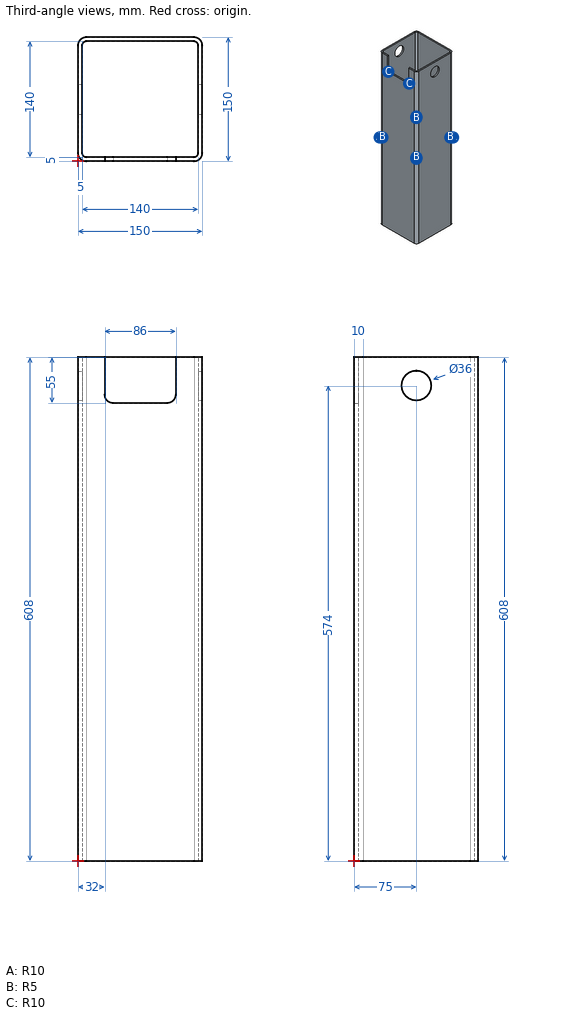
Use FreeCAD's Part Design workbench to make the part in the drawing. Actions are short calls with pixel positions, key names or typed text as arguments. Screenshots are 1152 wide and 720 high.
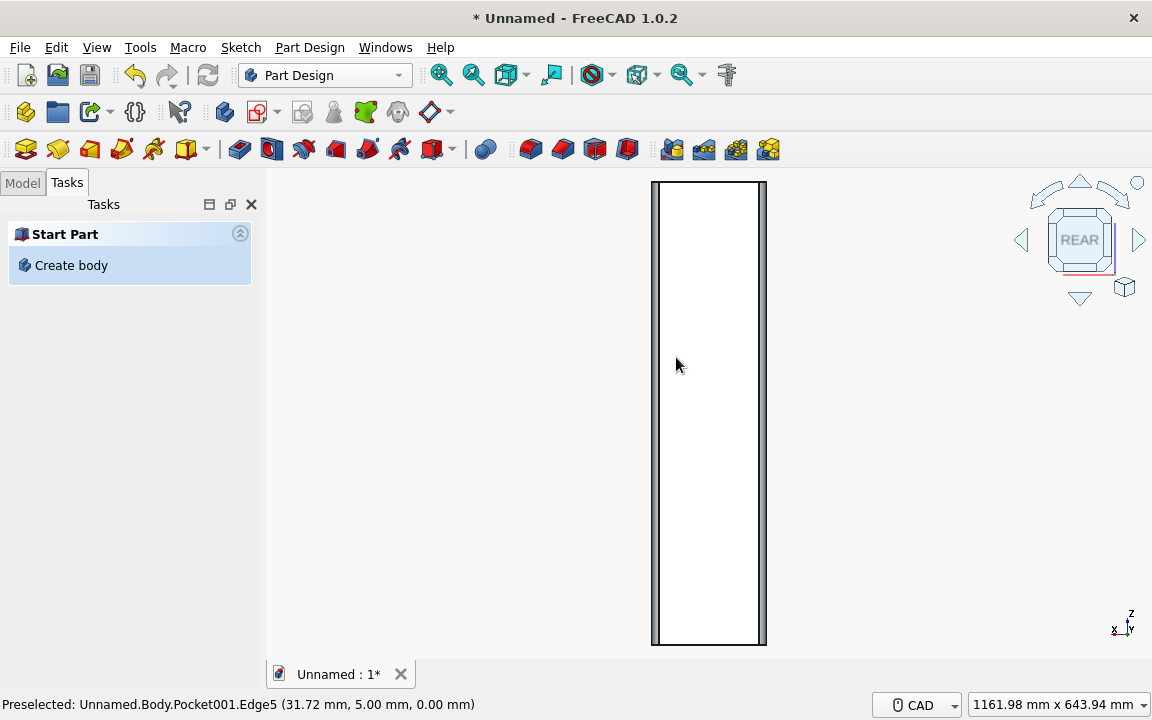
scroll(742, 223, up, 12)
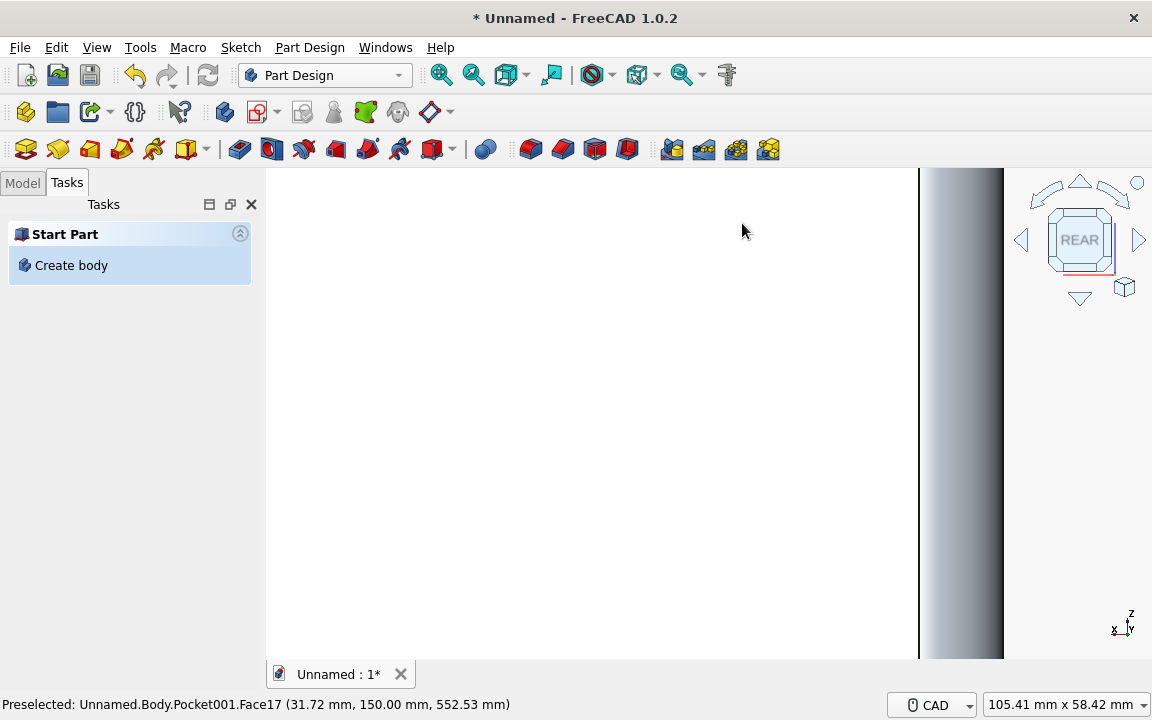
key(v)
key(f)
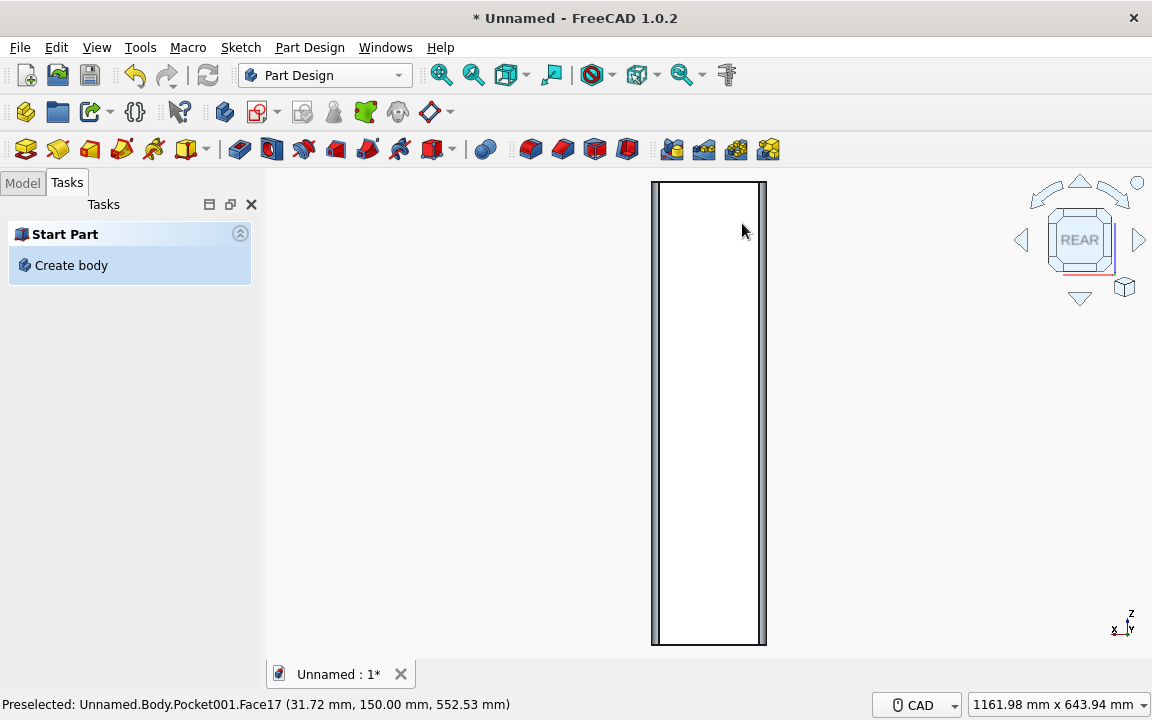
key(6)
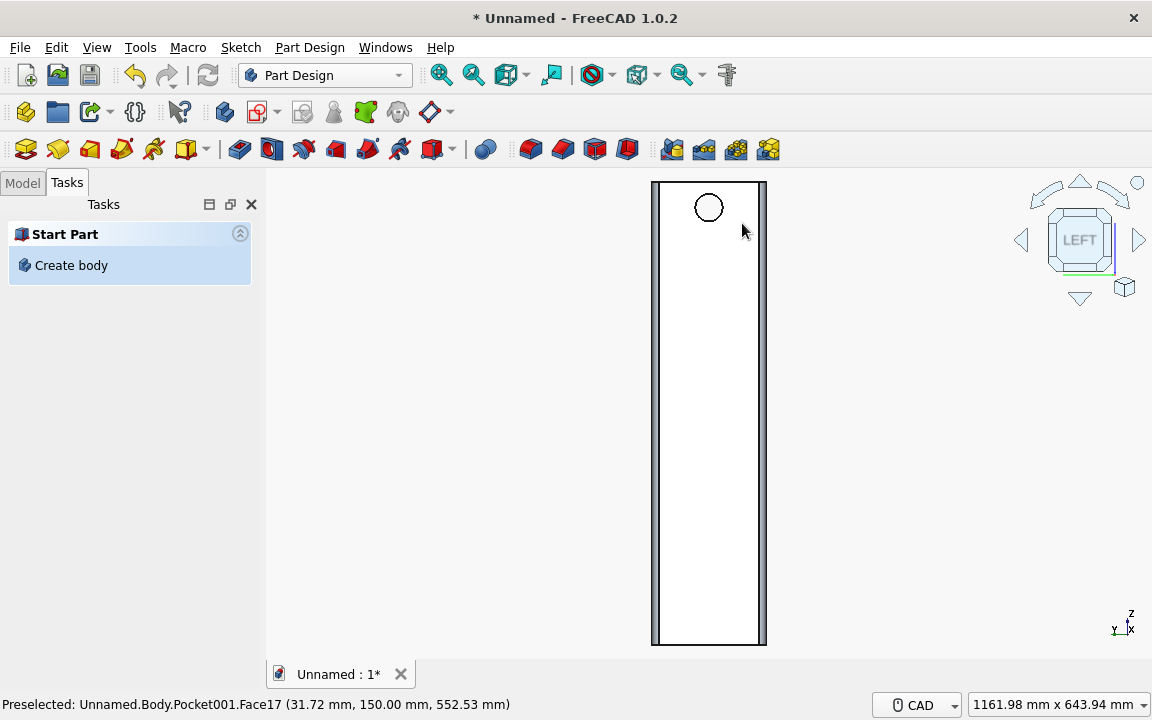
scroll(764, 223, up, 12)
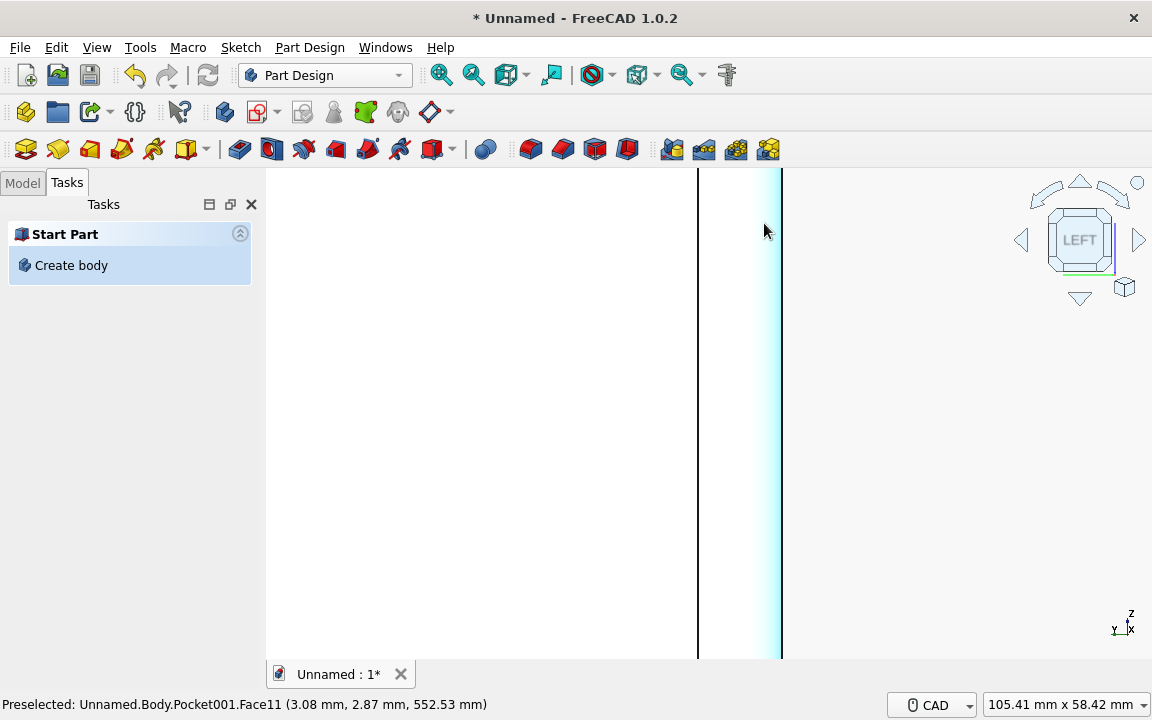
key(v)
key(f)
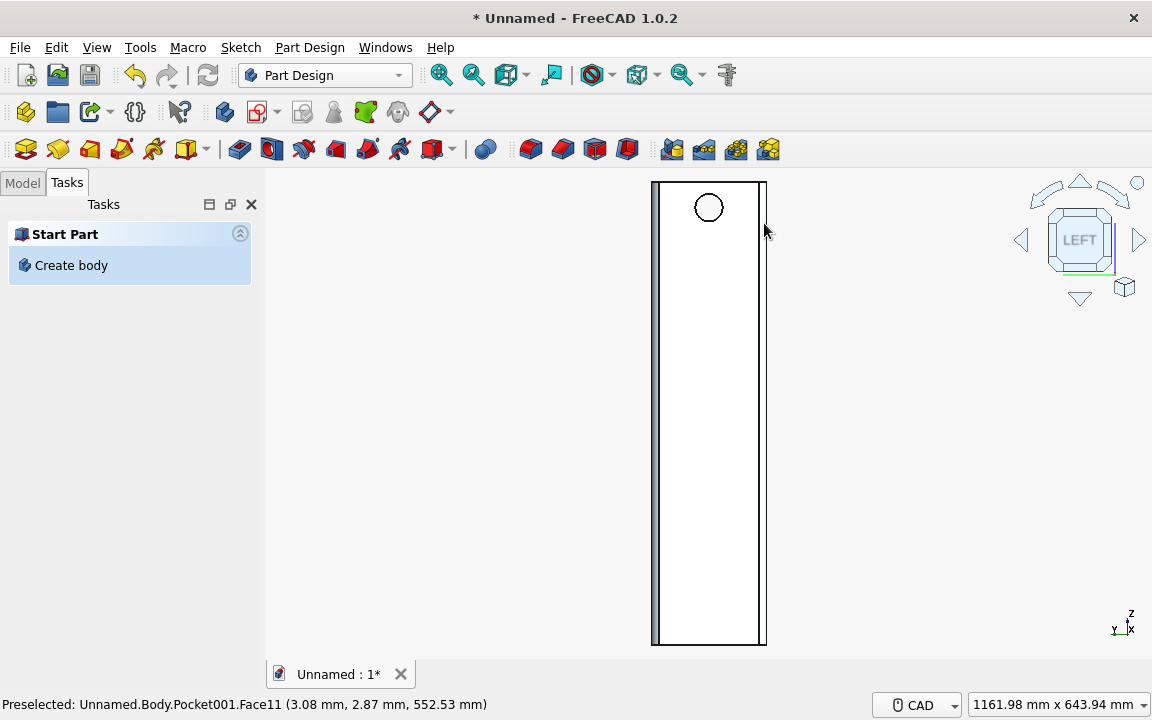
key(v)
key(3)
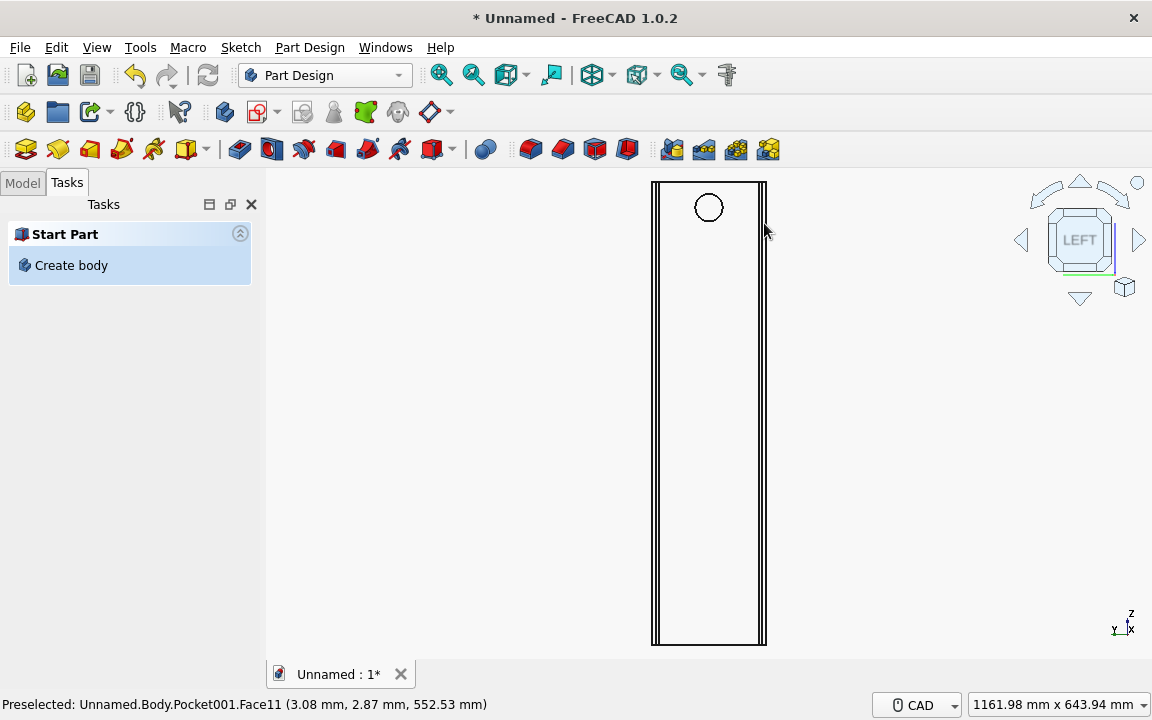
key(0)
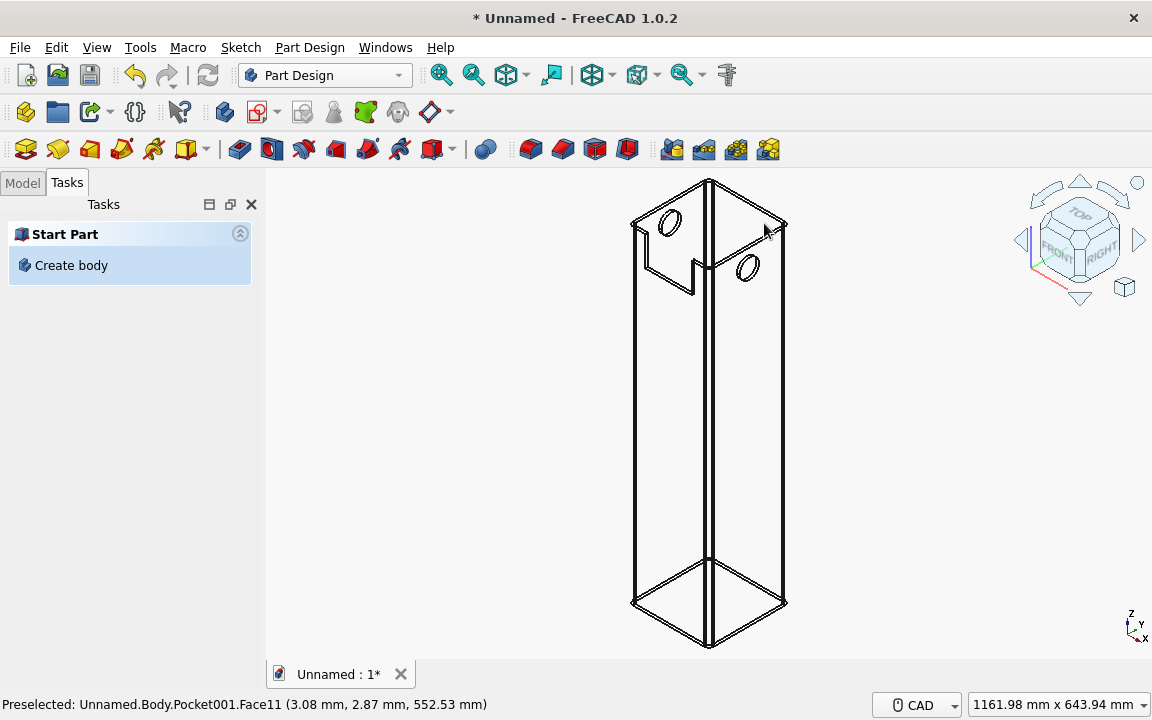
scroll(647, 267, up, 12)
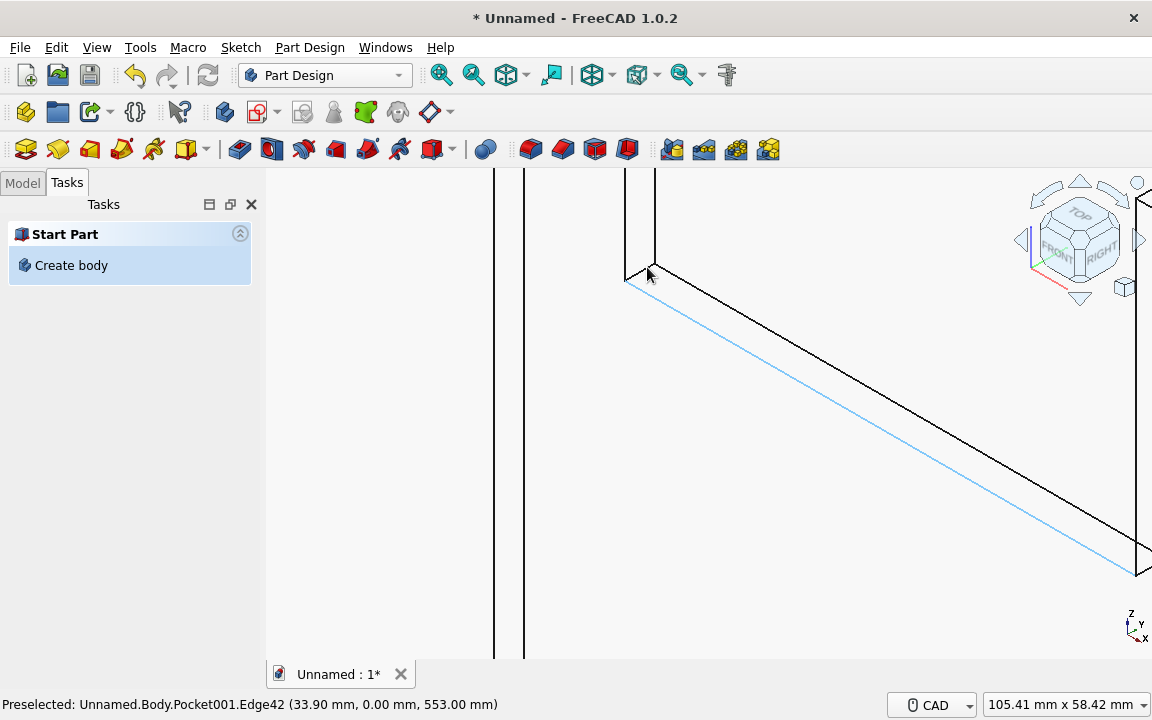
click(640, 271)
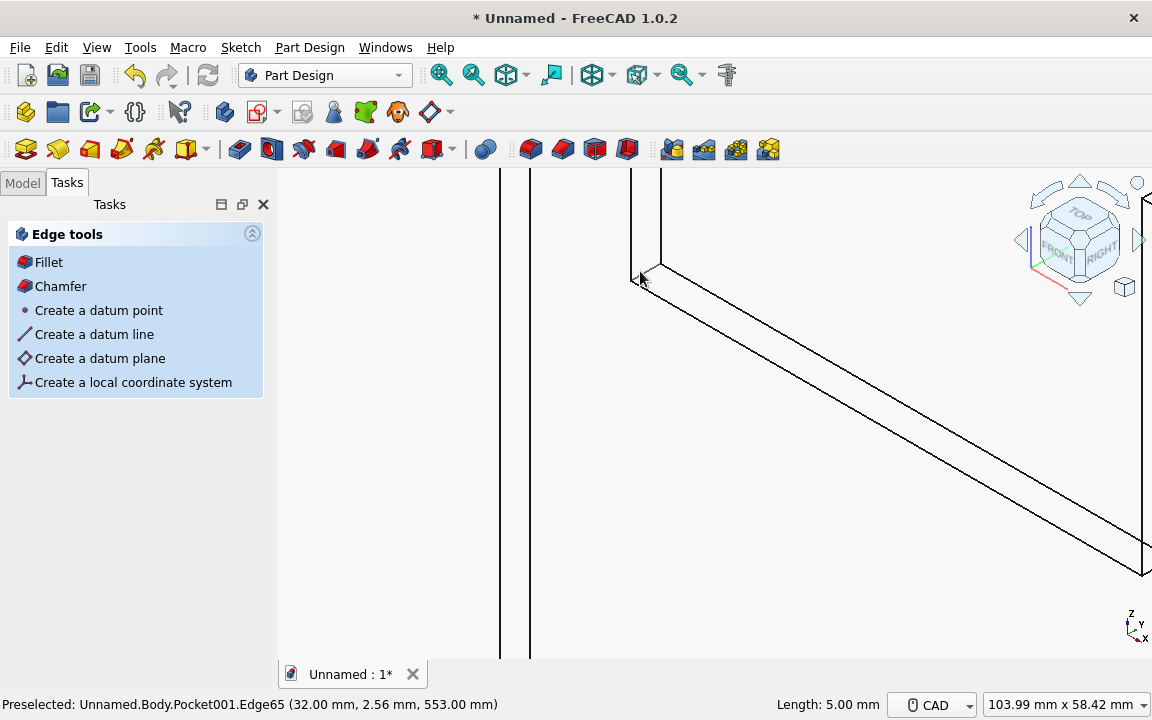
key(v)
key(f)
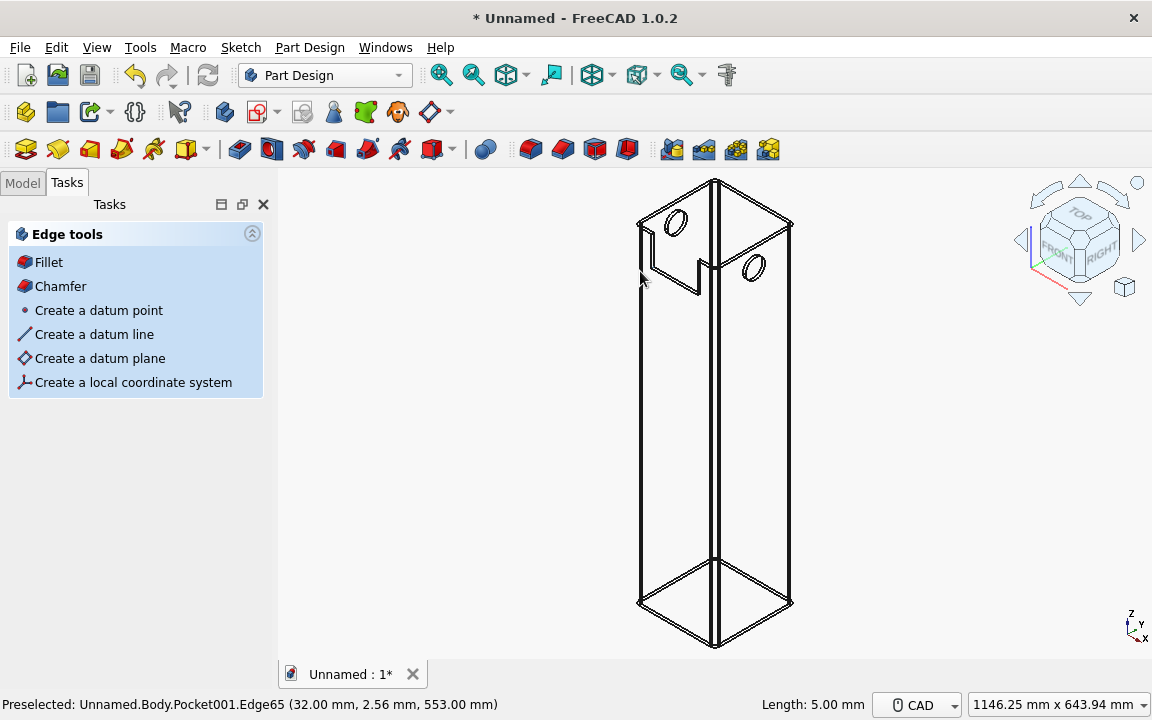
key(2)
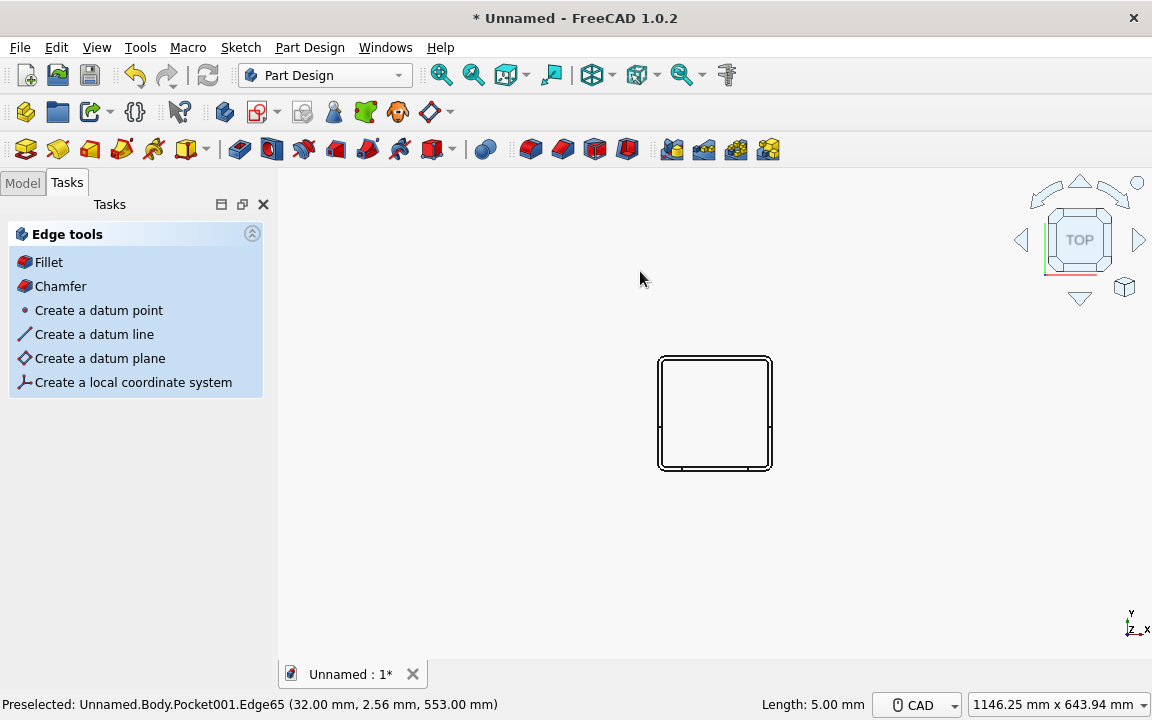
click(442, 76)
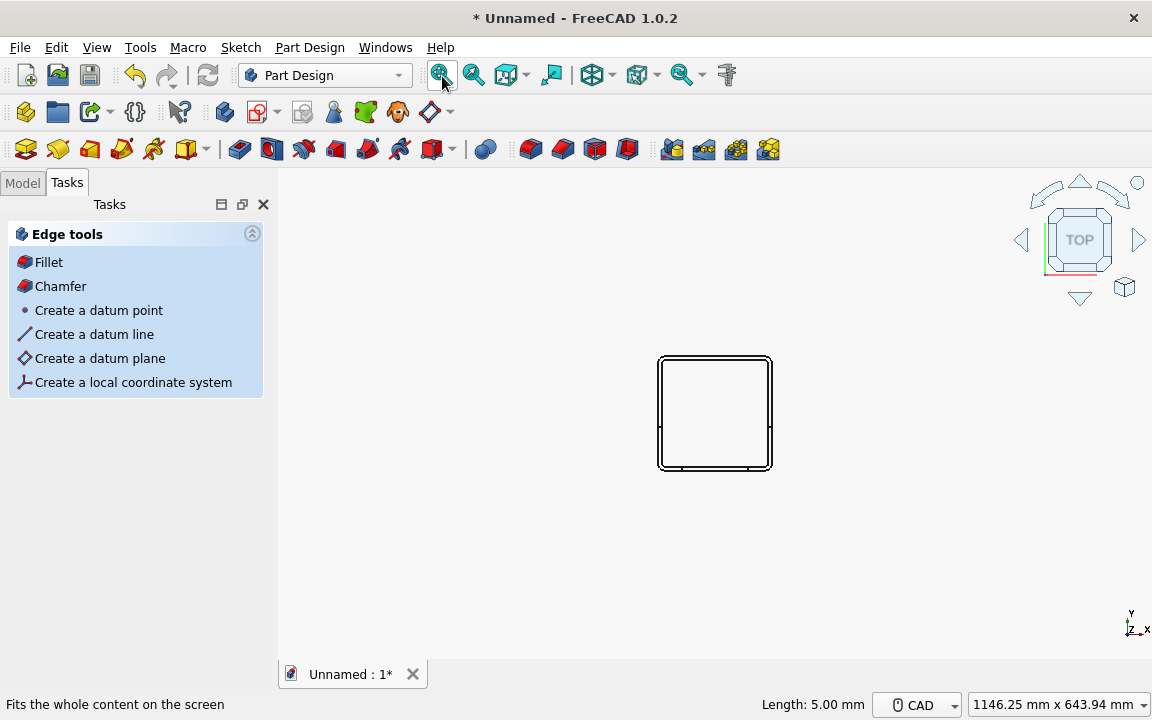
scroll(748, 468, up, 12)